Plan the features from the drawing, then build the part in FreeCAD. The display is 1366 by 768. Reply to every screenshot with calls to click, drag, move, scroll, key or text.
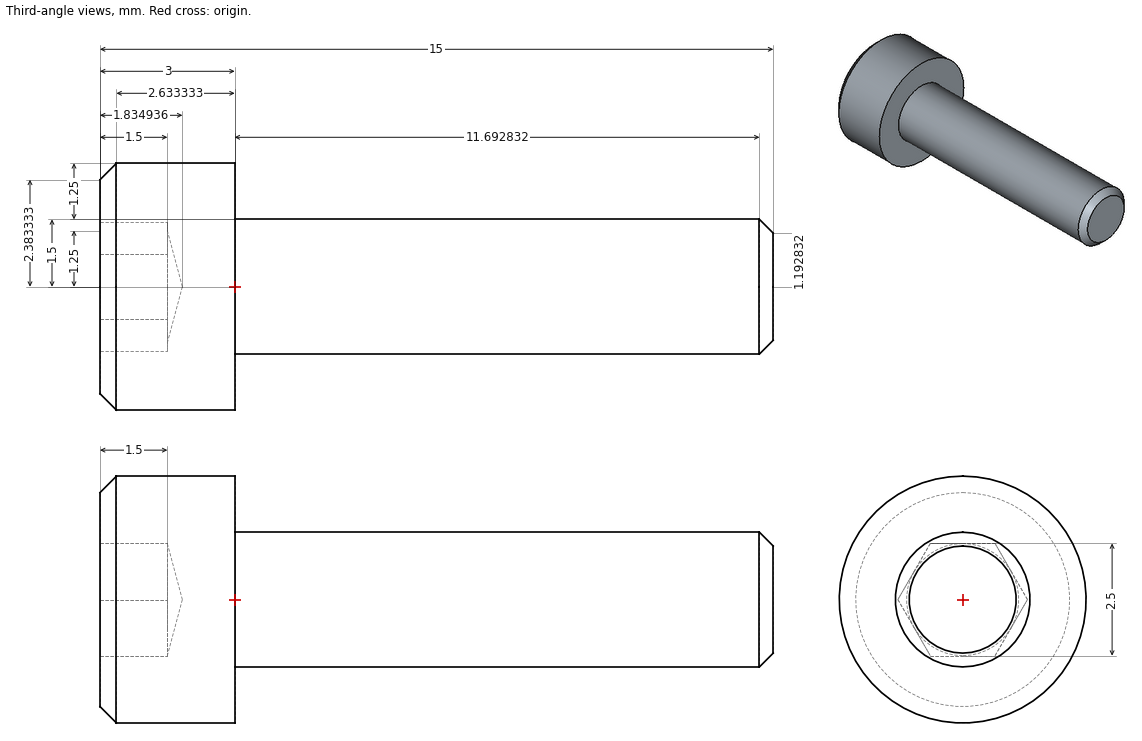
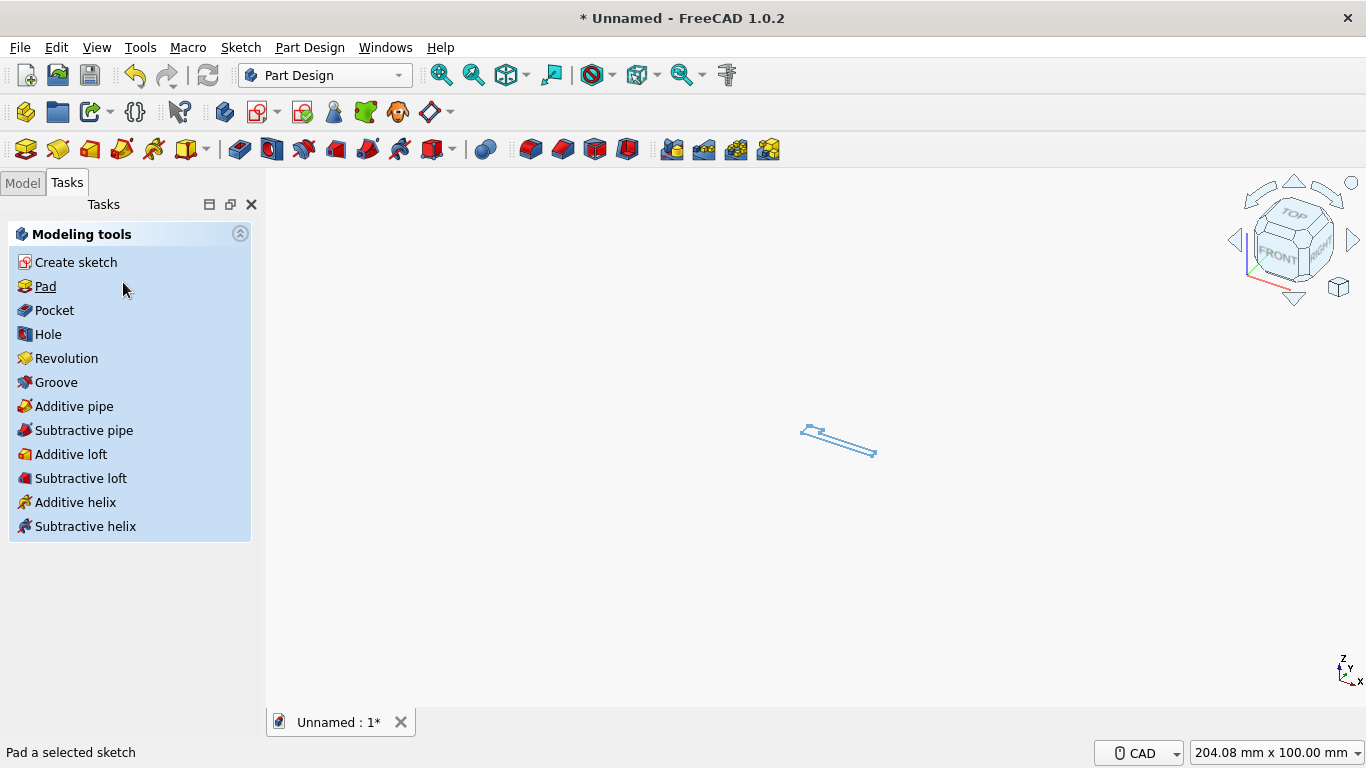
click(58, 150)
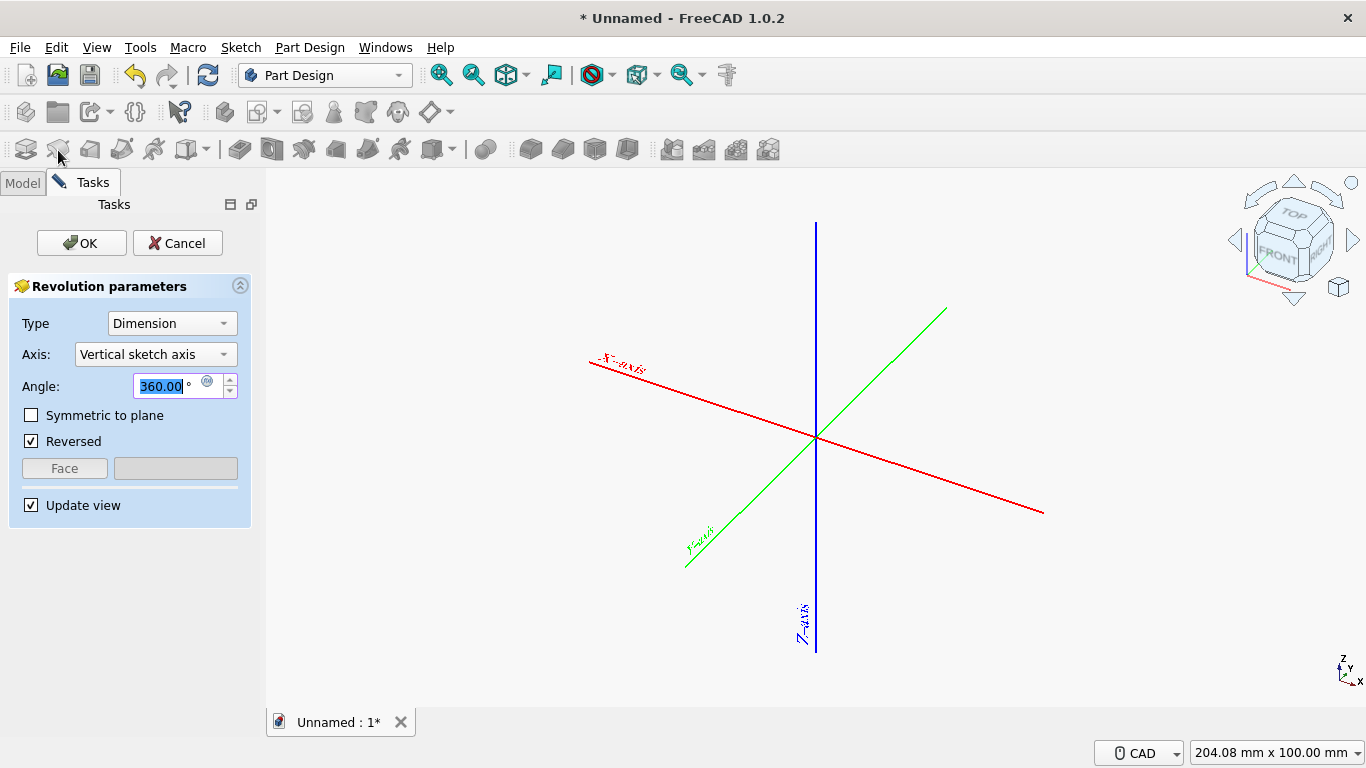
click(156, 354)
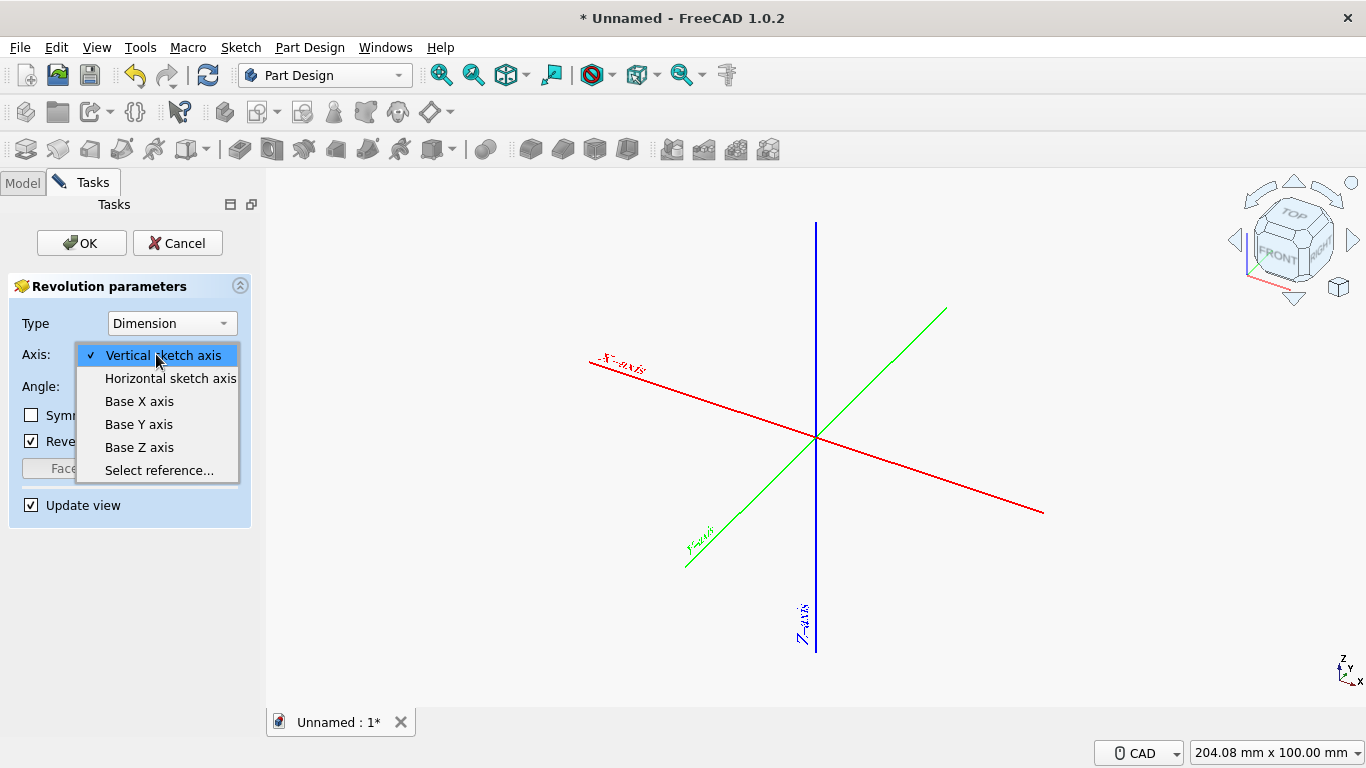
click(156, 378)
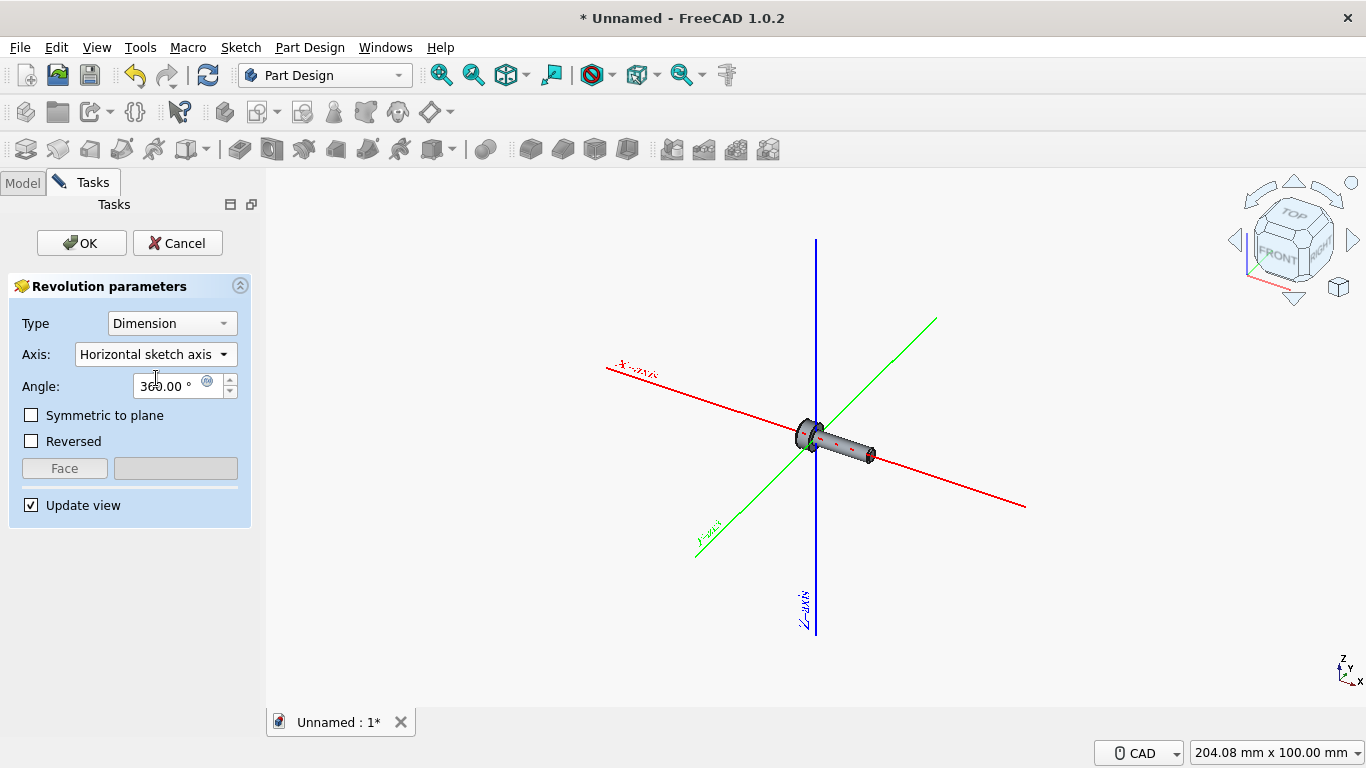
click(82, 243)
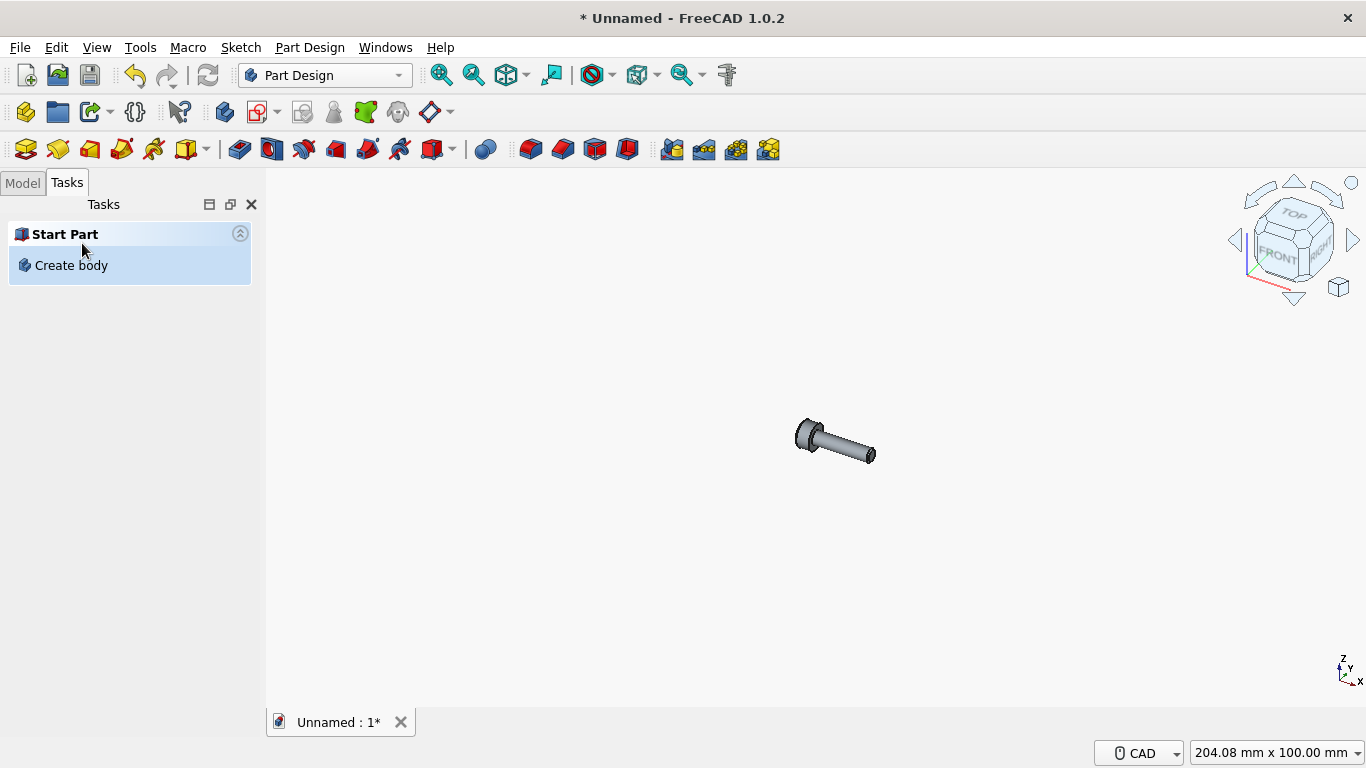
click(442, 76)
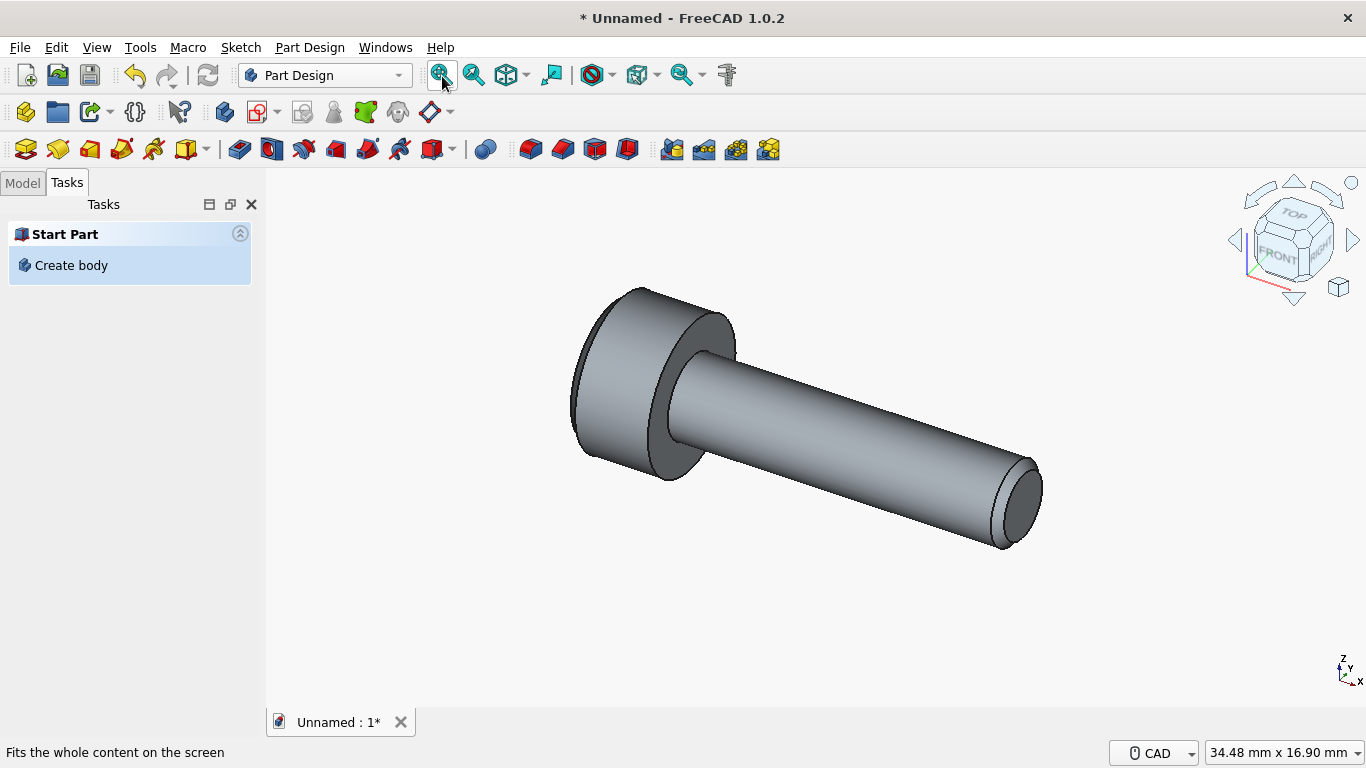
click(258, 112)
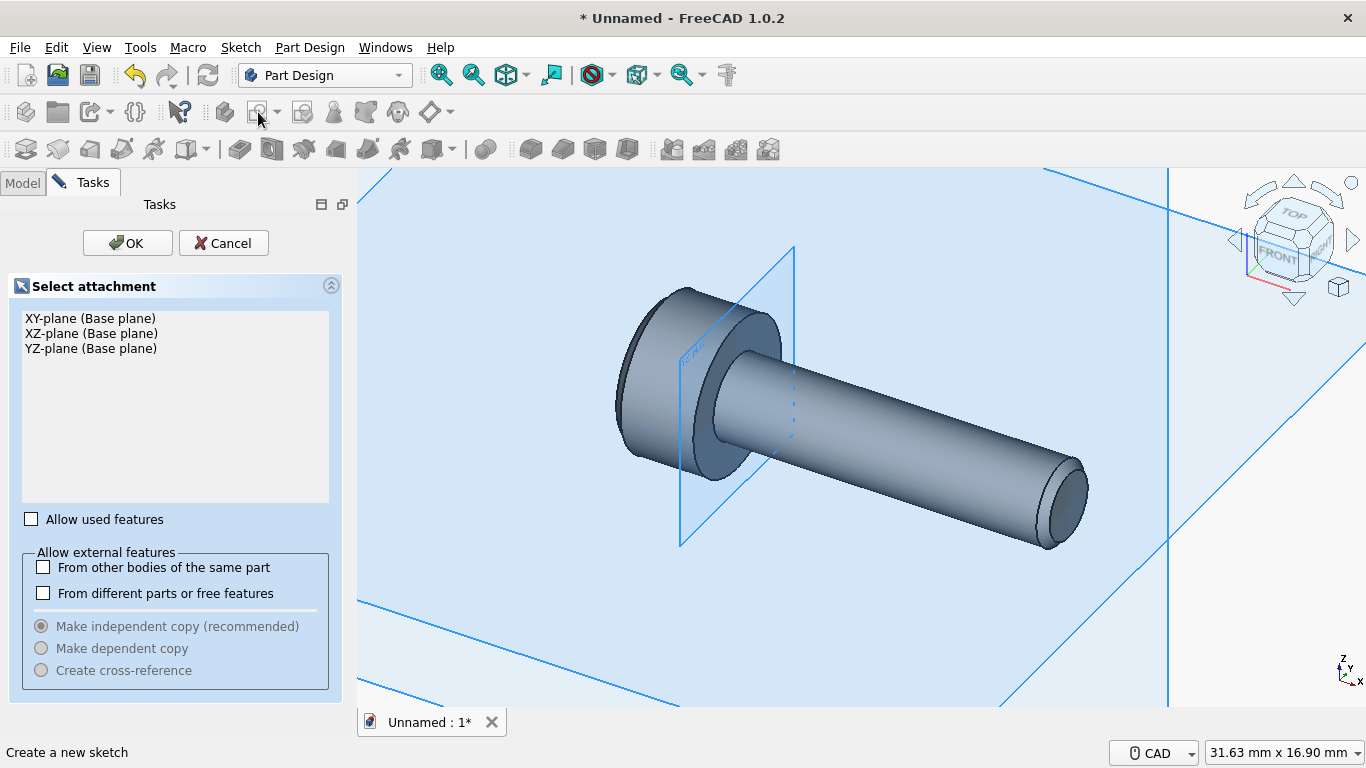
click(82, 318)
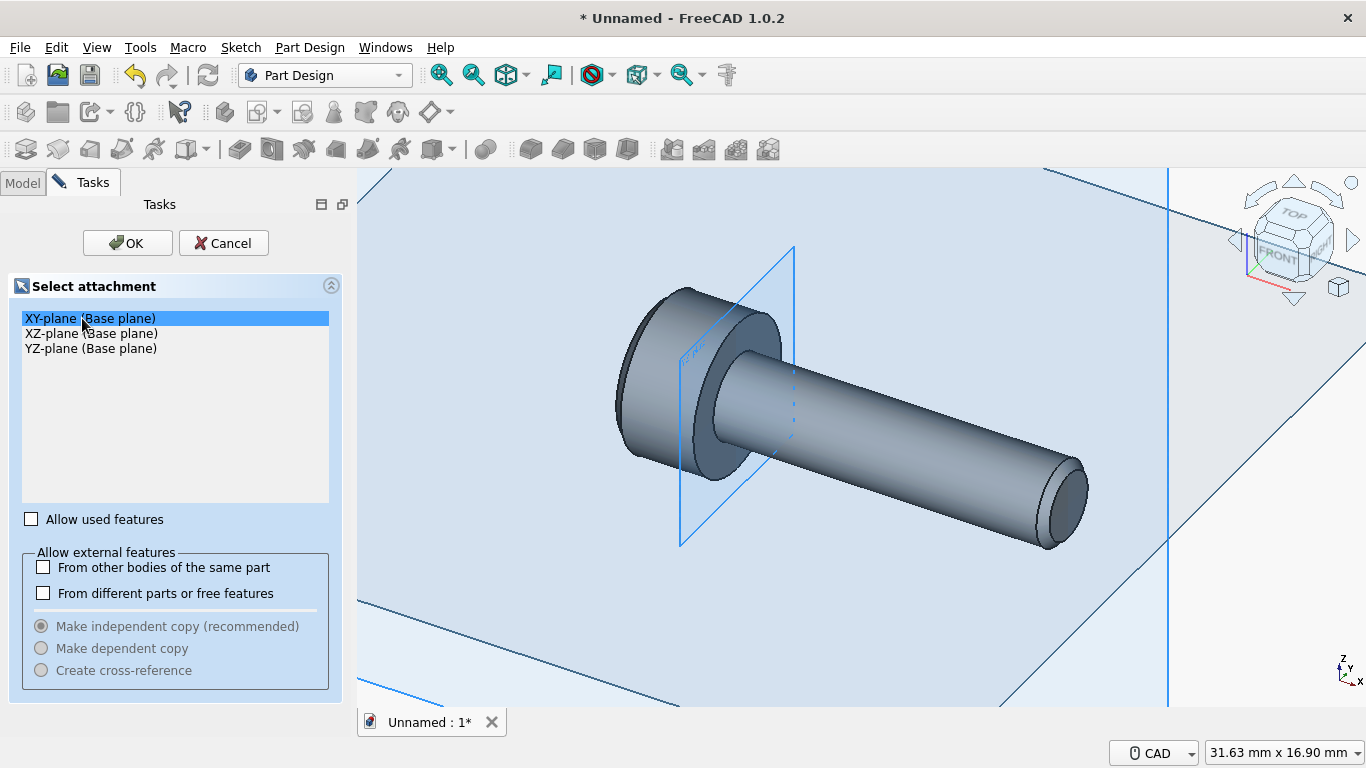
click(128, 243)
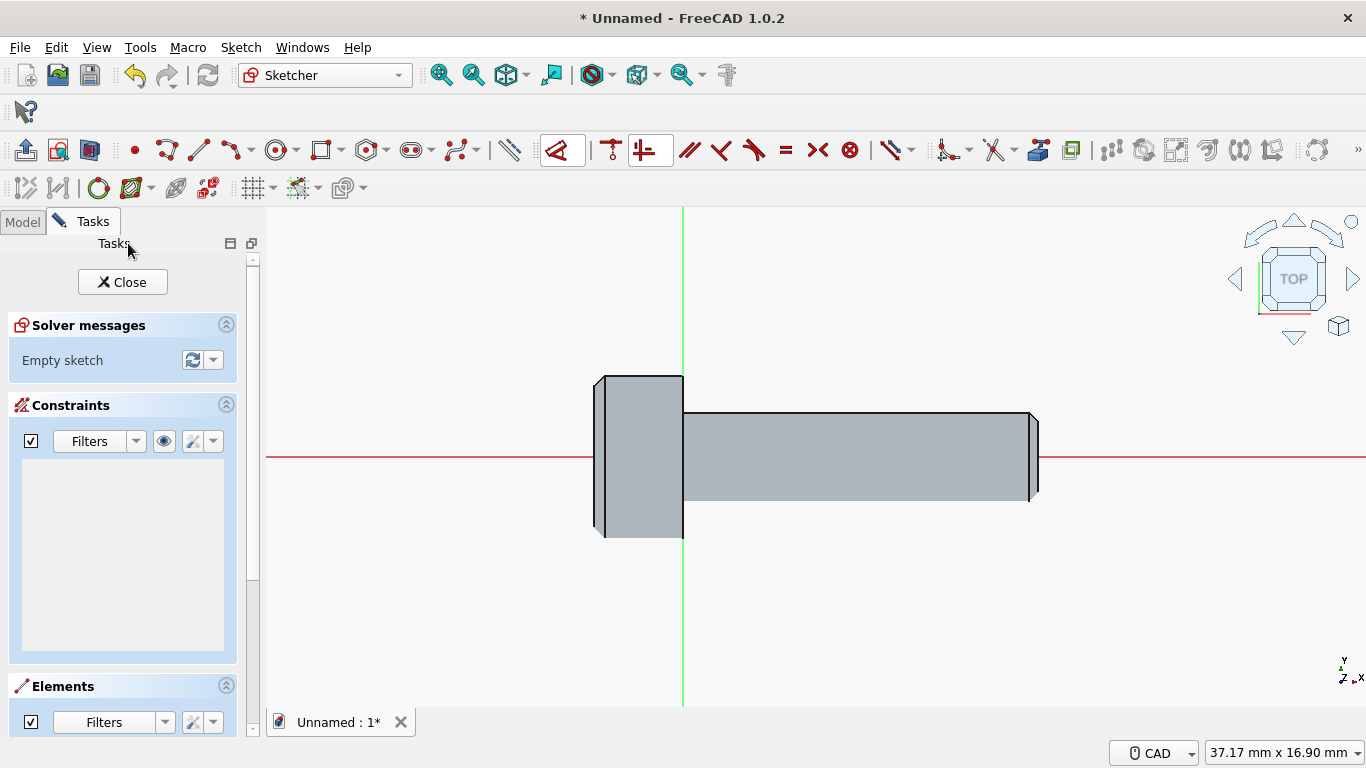
click(90, 150)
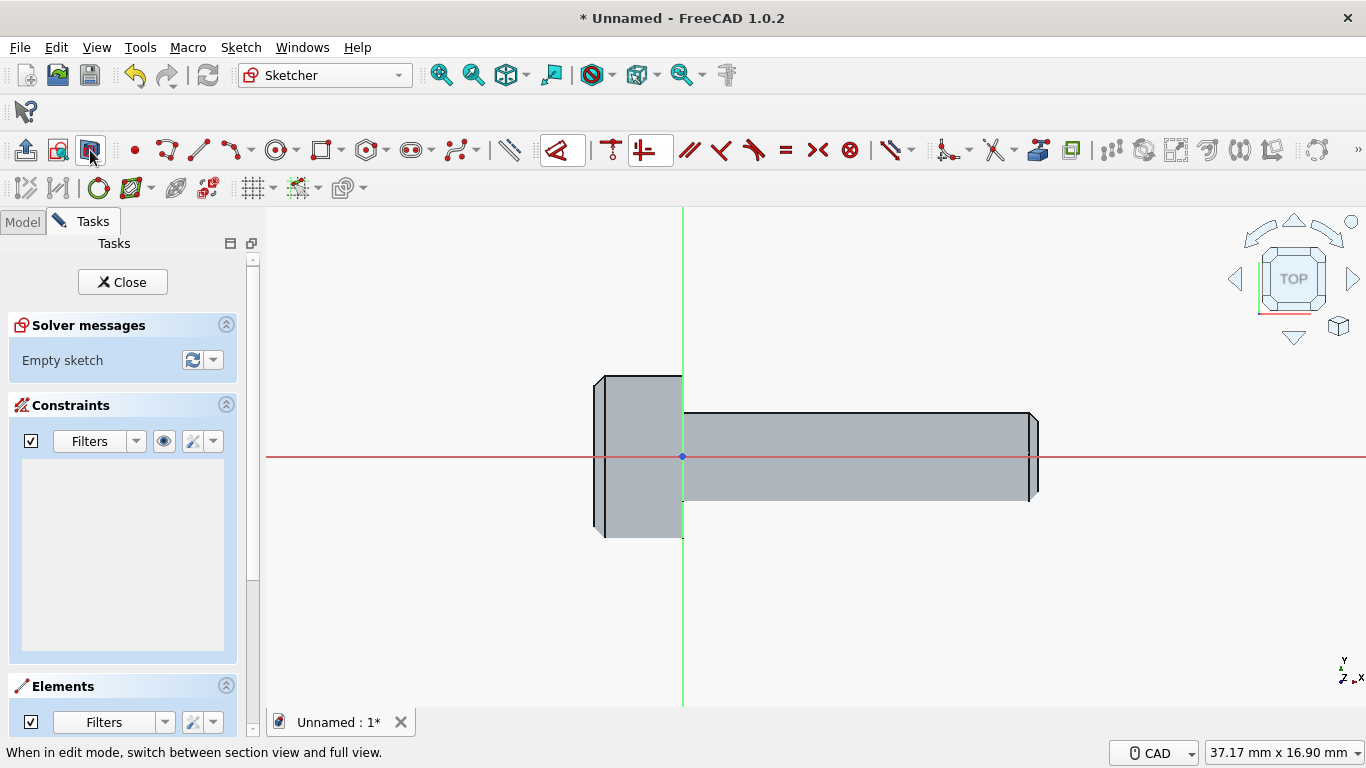
scroll(621, 436, up, 10)